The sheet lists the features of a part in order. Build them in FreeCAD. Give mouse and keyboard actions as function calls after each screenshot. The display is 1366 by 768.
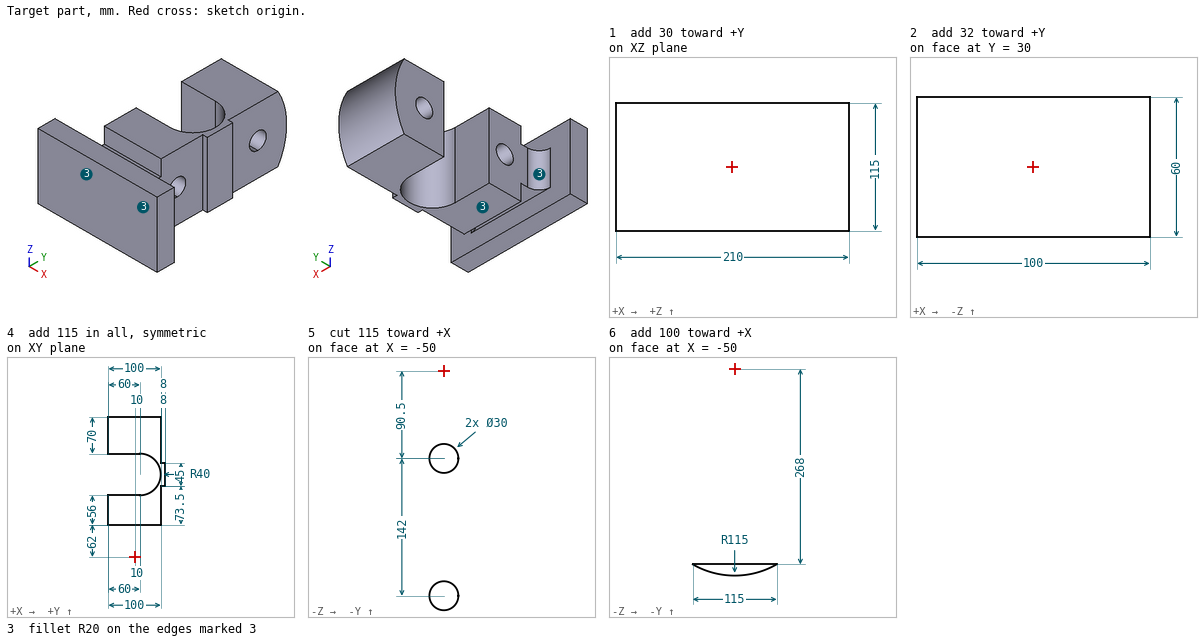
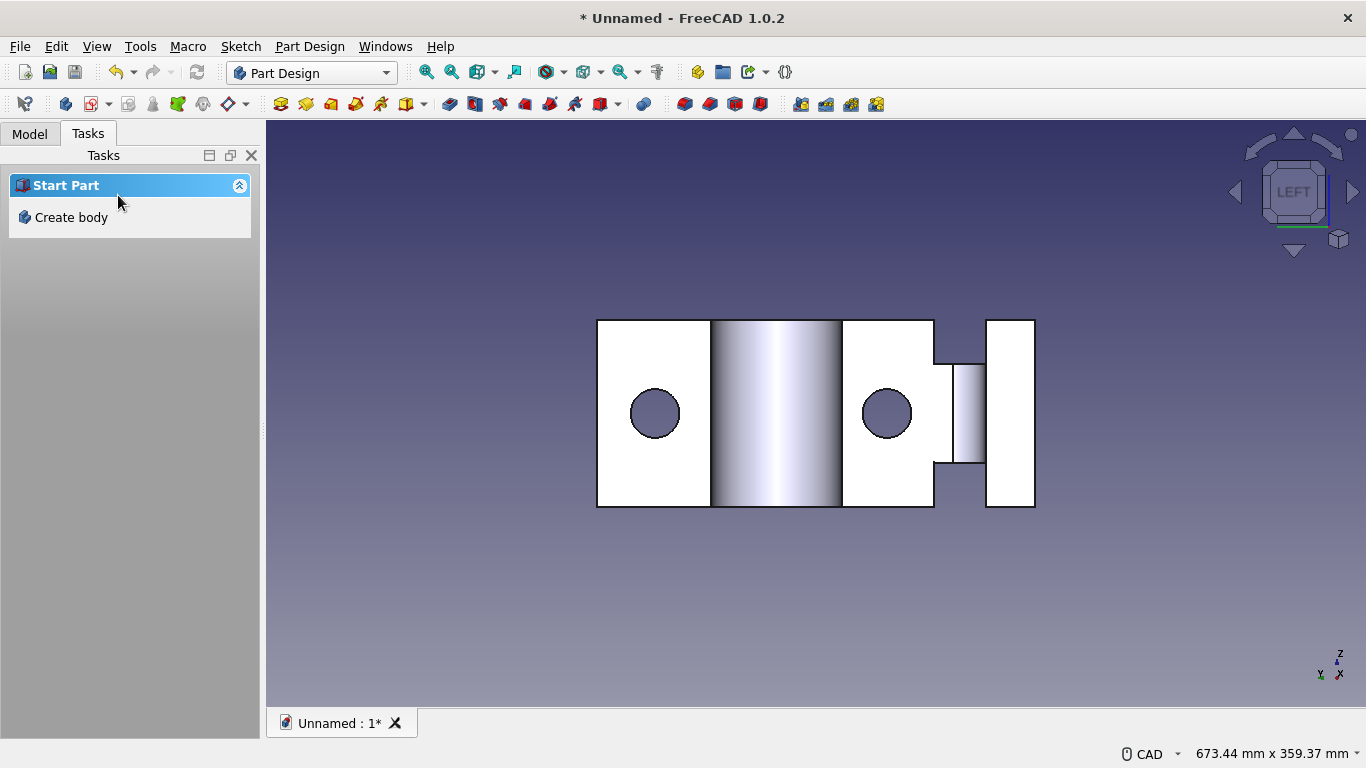
click(638, 359)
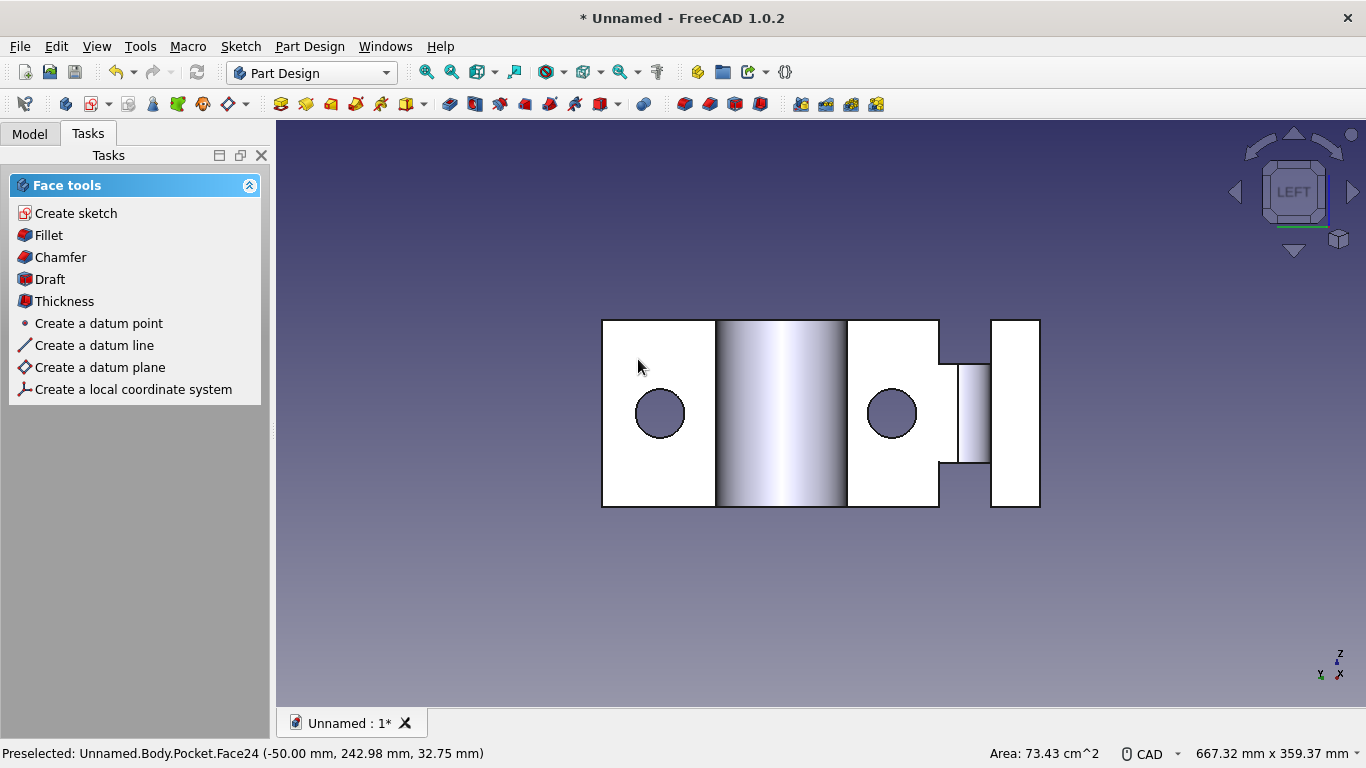
click(90, 104)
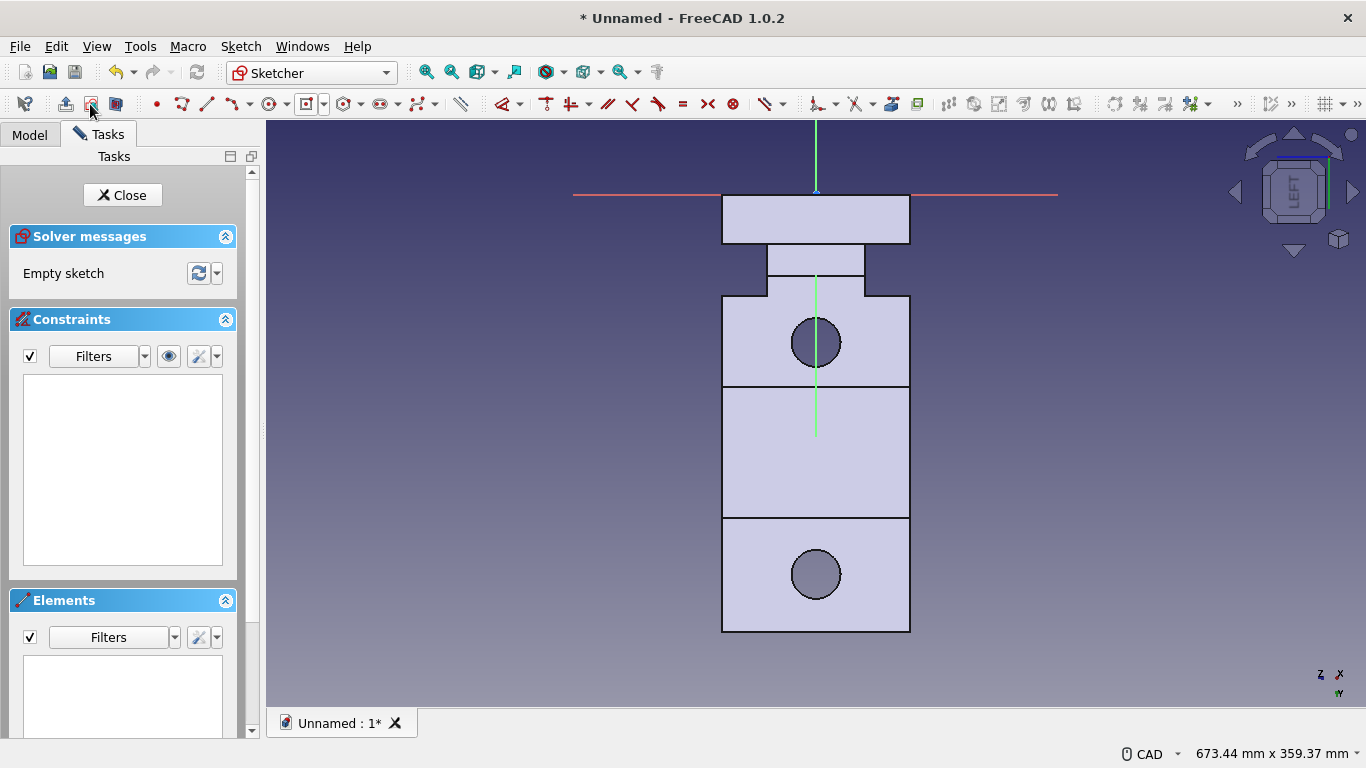
key(q)
key(s)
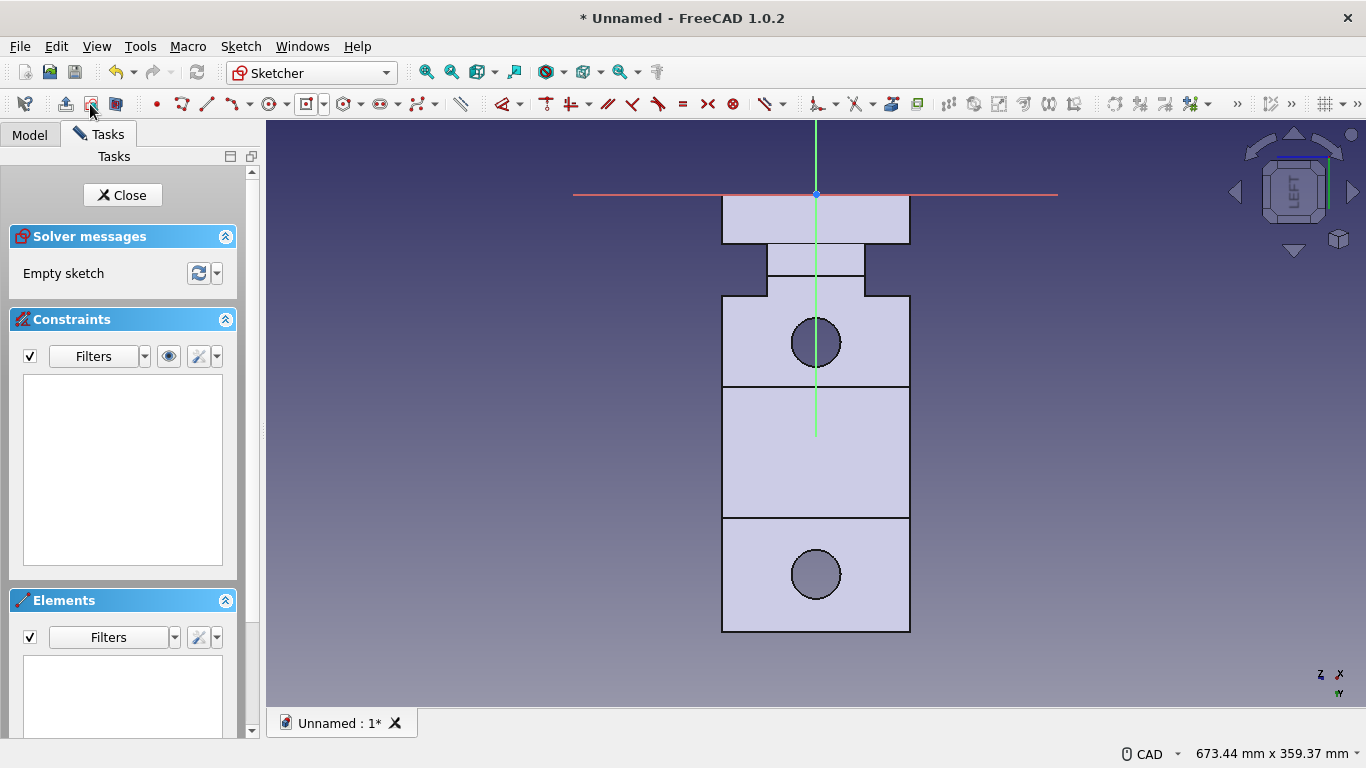
scroll(438, 357, down, 1)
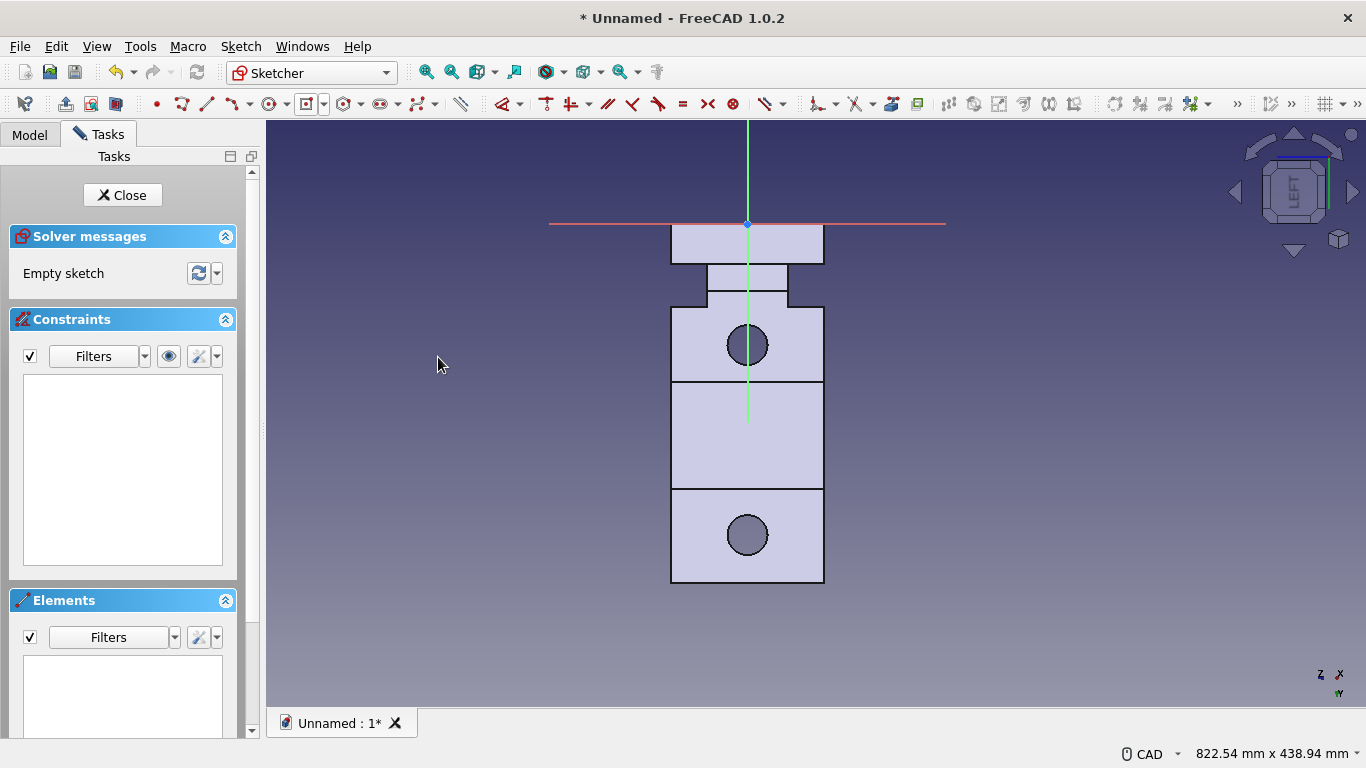
key(g)
key(l)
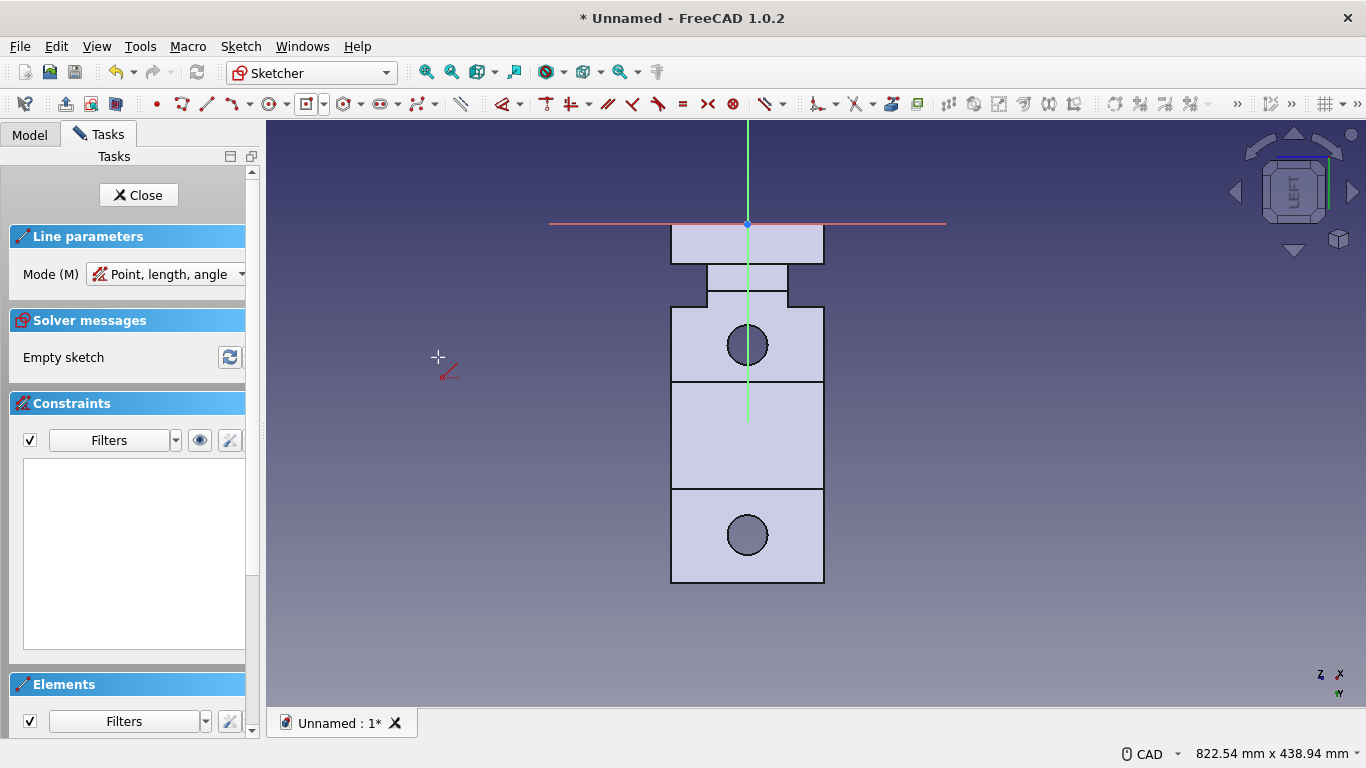
click(824, 583)
click(671, 583)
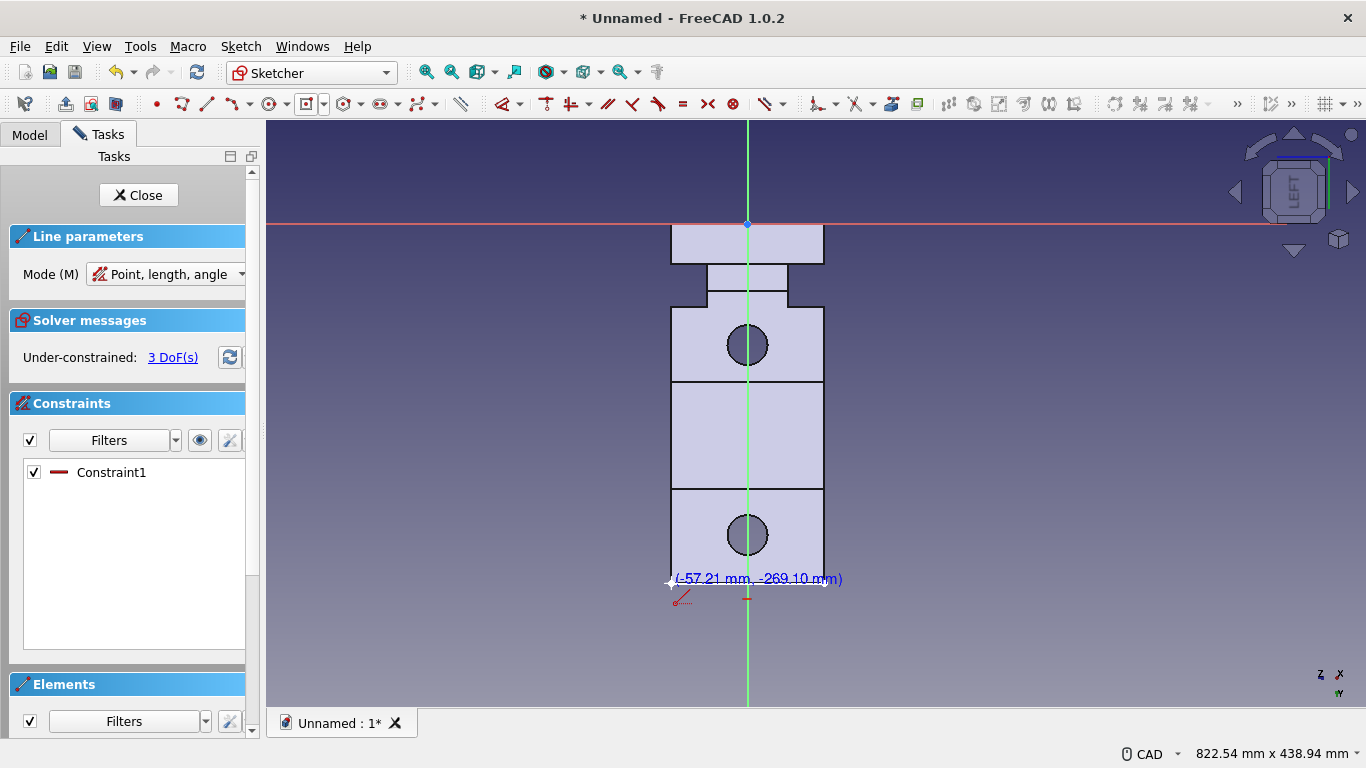
key(g)
key(3)
key(a)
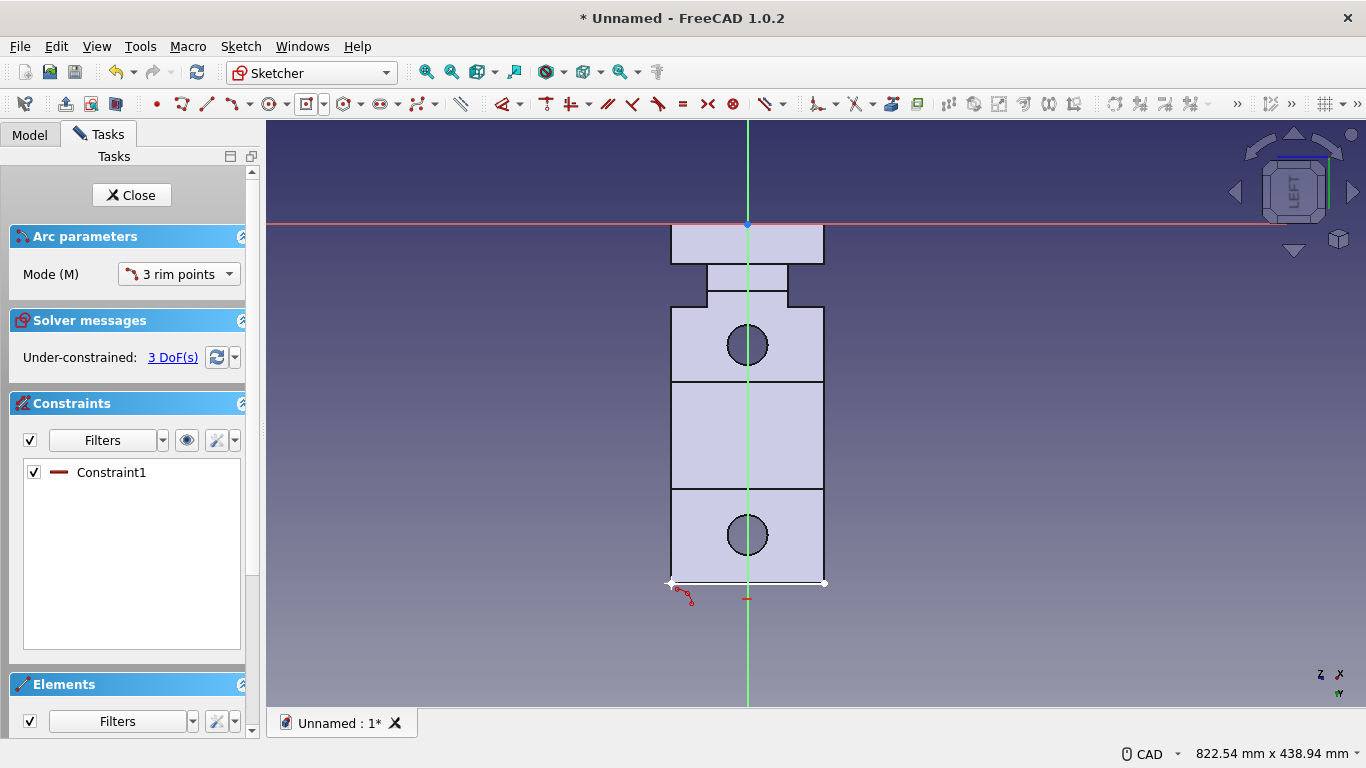
click(671, 584)
click(824, 584)
click(731, 602)
key(Escape)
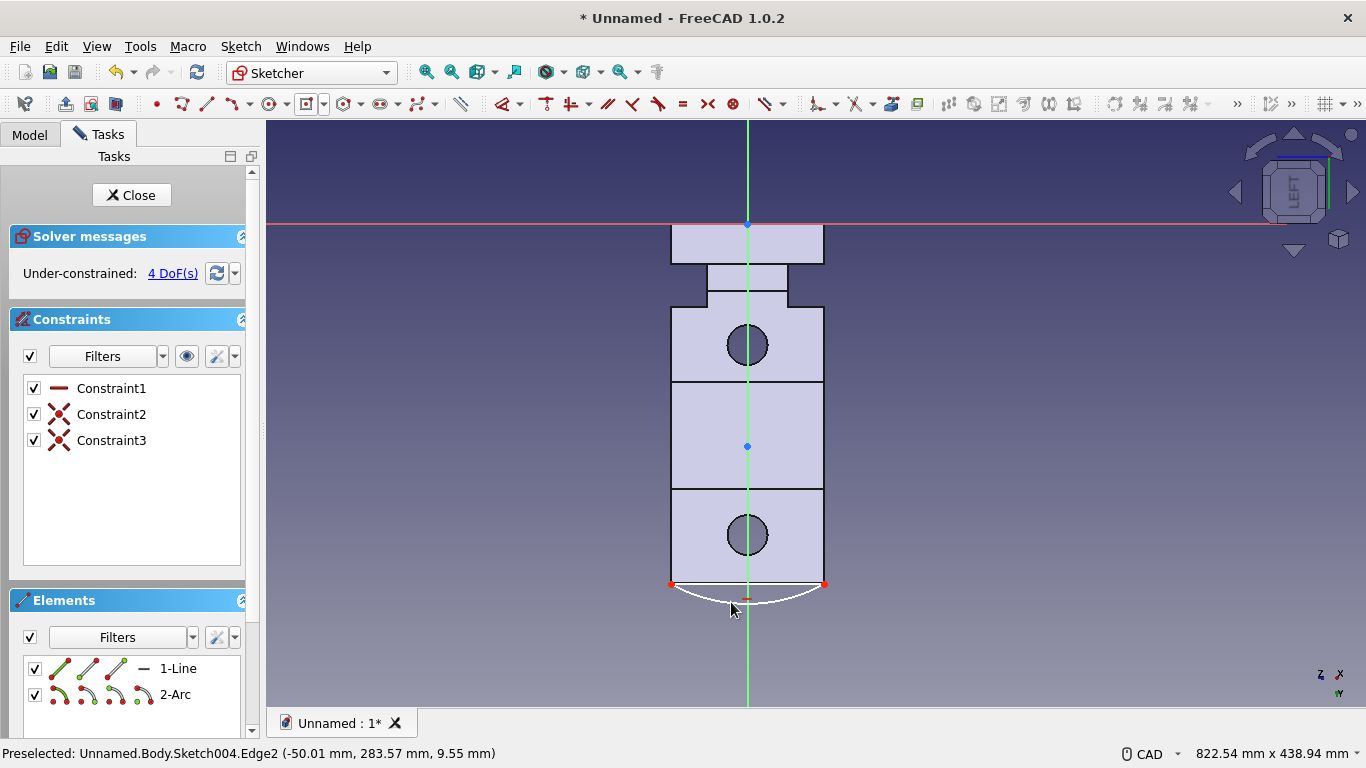
click(747, 447)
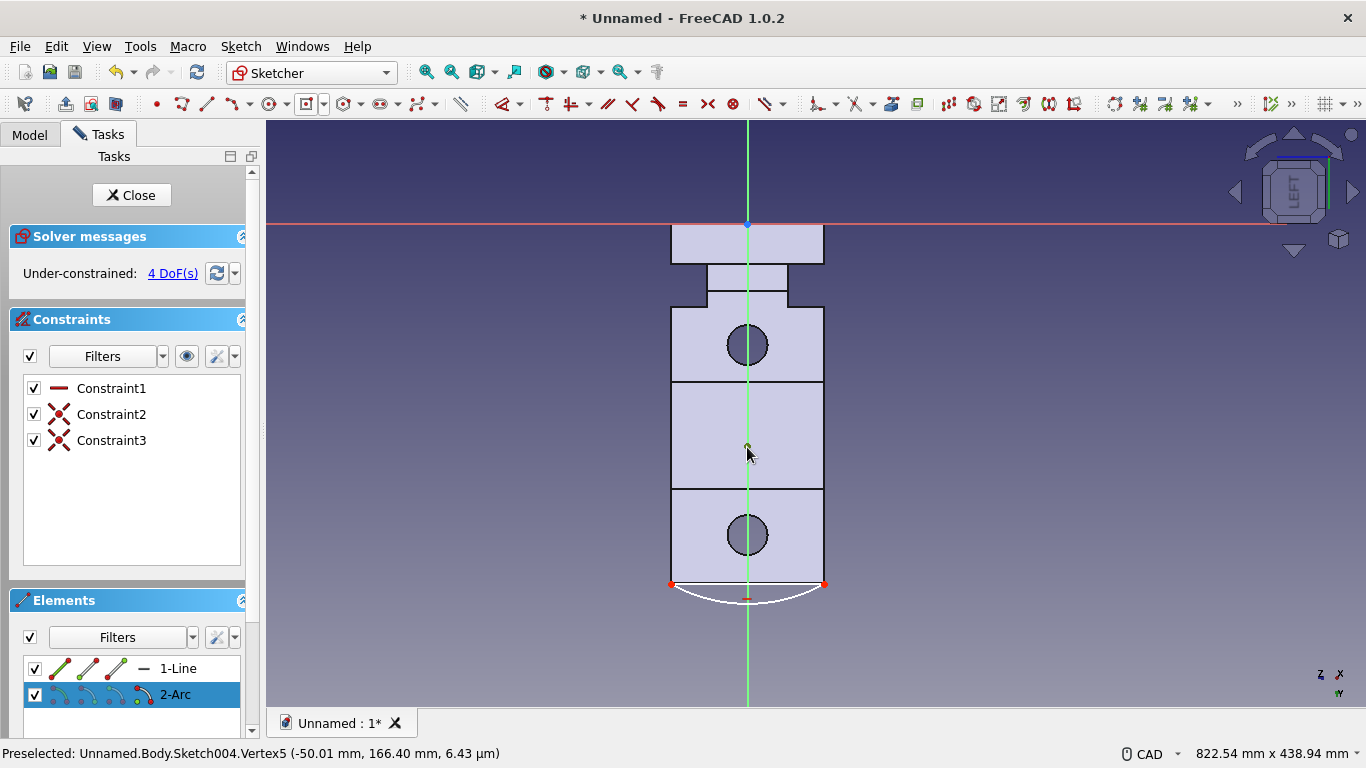
click(748, 641)